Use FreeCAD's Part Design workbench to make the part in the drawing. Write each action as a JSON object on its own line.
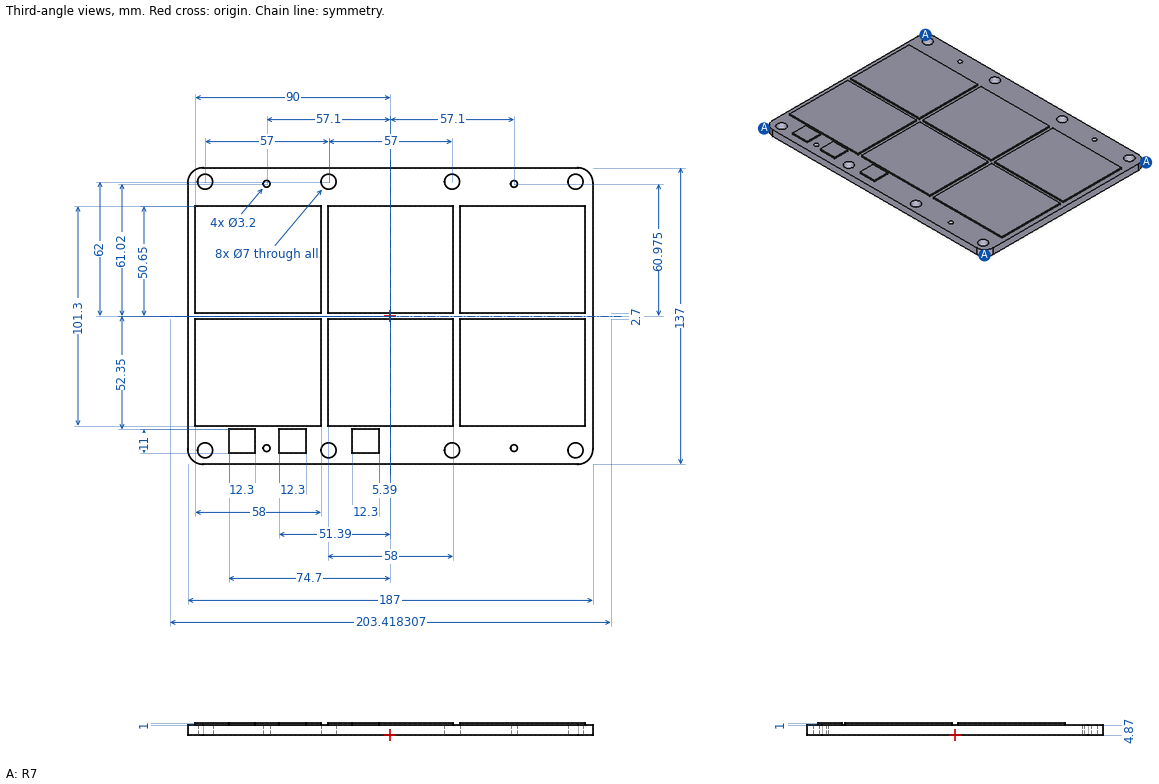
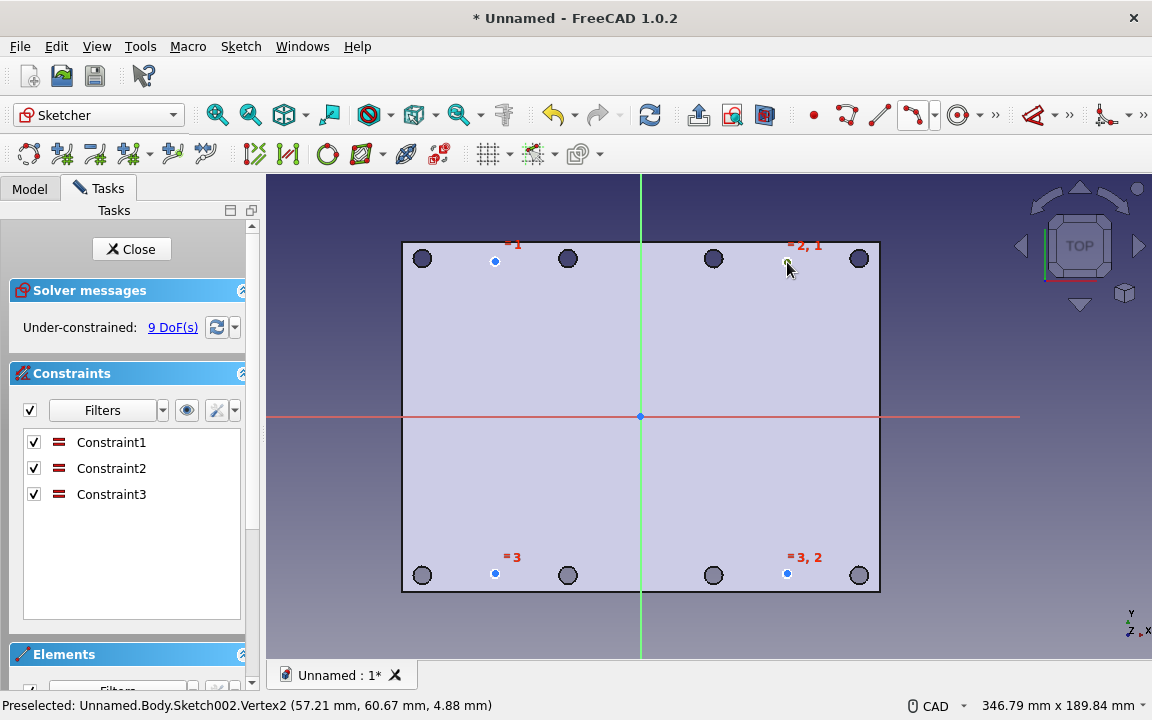
{"action": "left_click", "coordinate": [787, 574]}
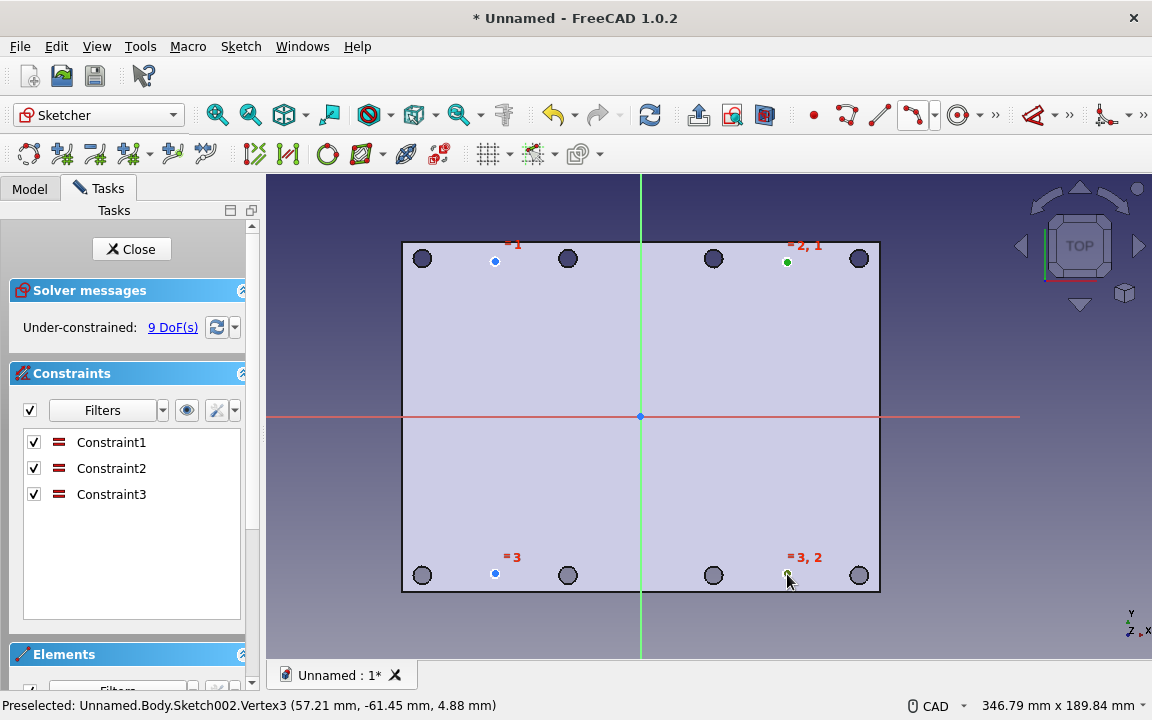
{"action": "left_click", "coordinate": [344, 417]}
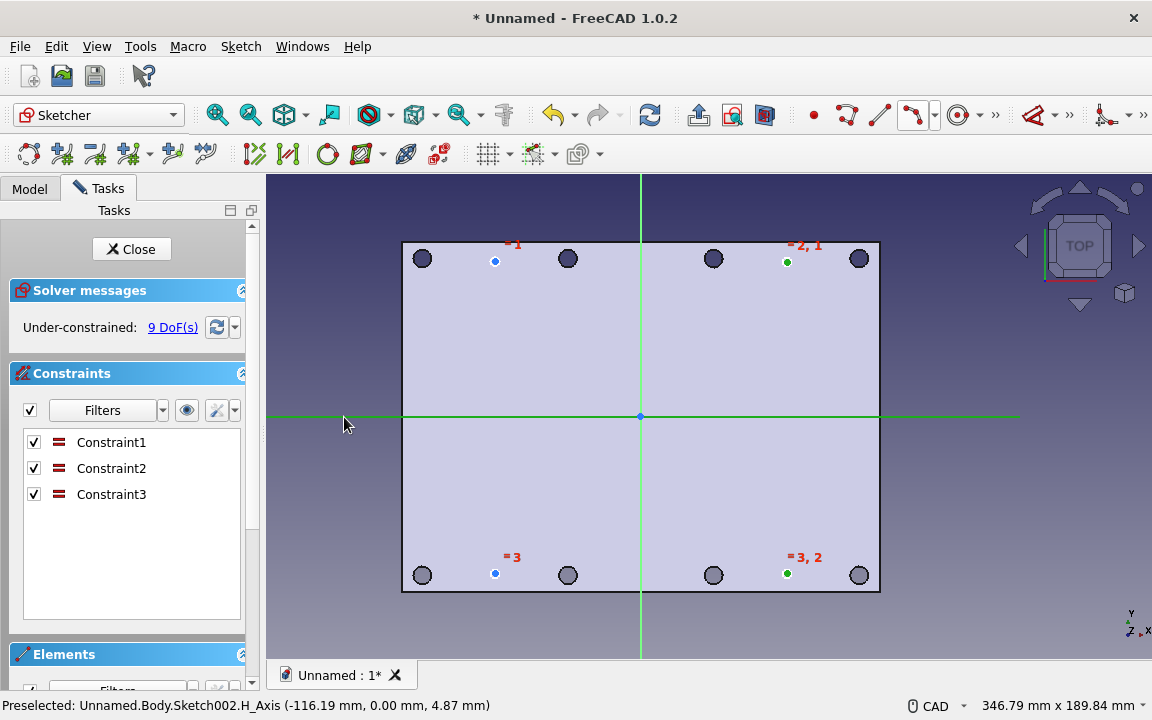
{"action": "key", "text": "s"}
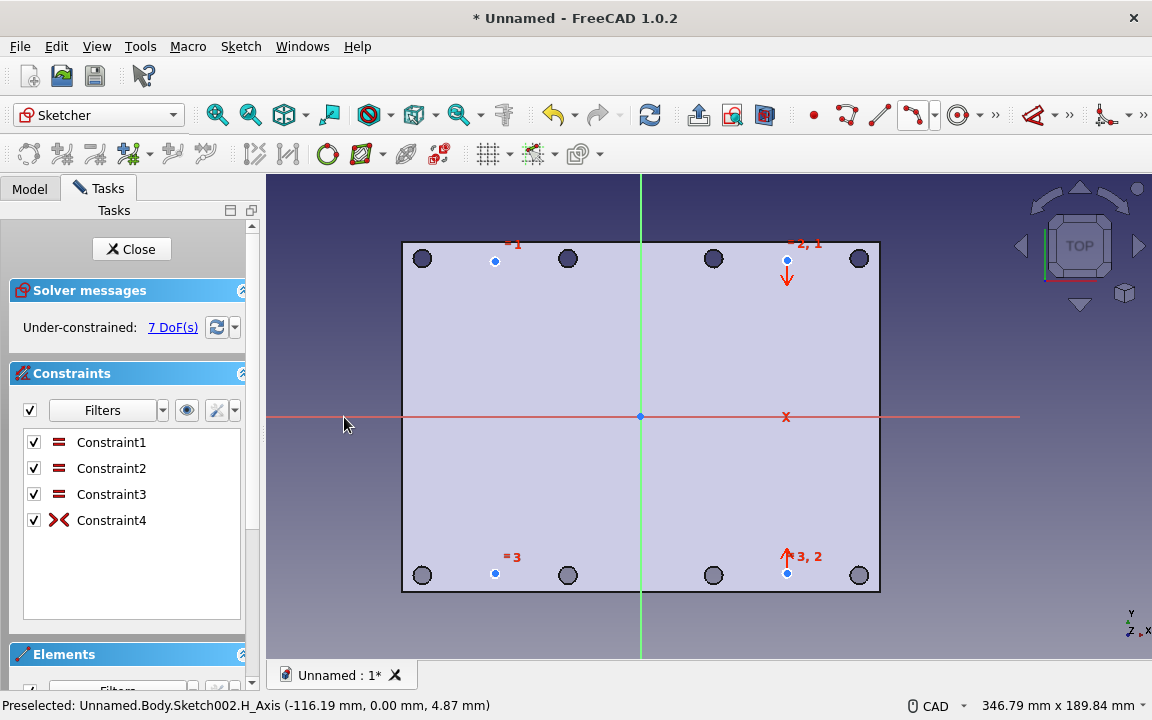
{"action": "left_click", "coordinate": [495, 262]}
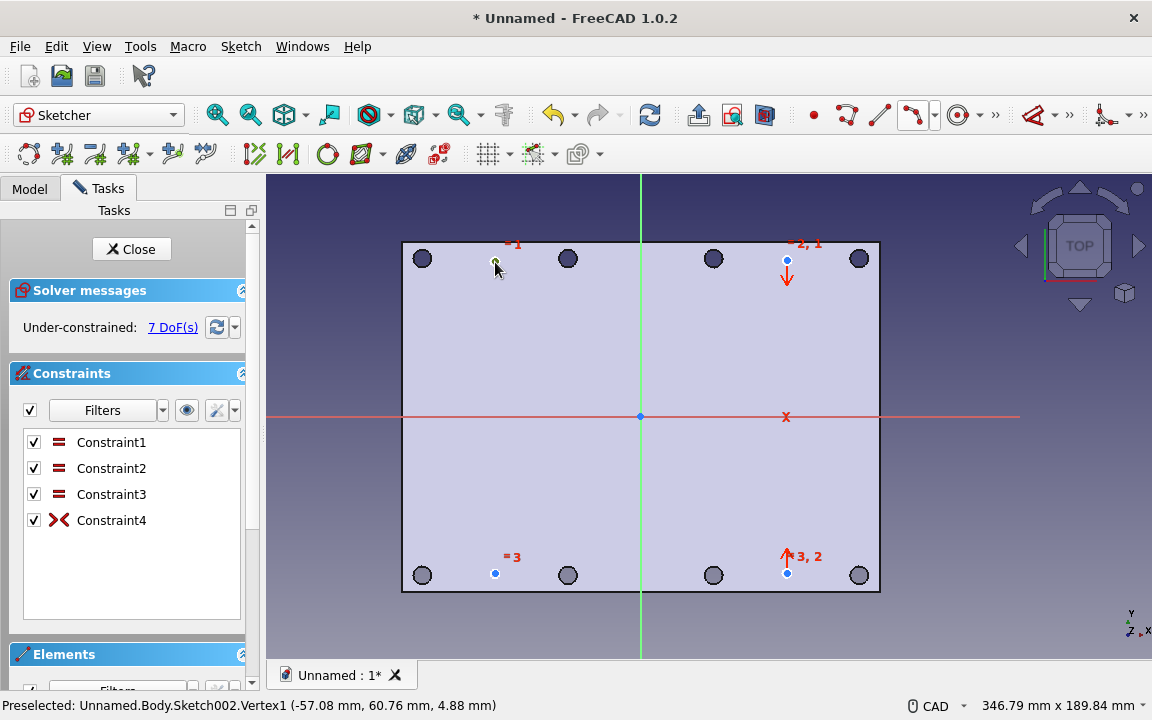
{"action": "left_click", "coordinate": [495, 574]}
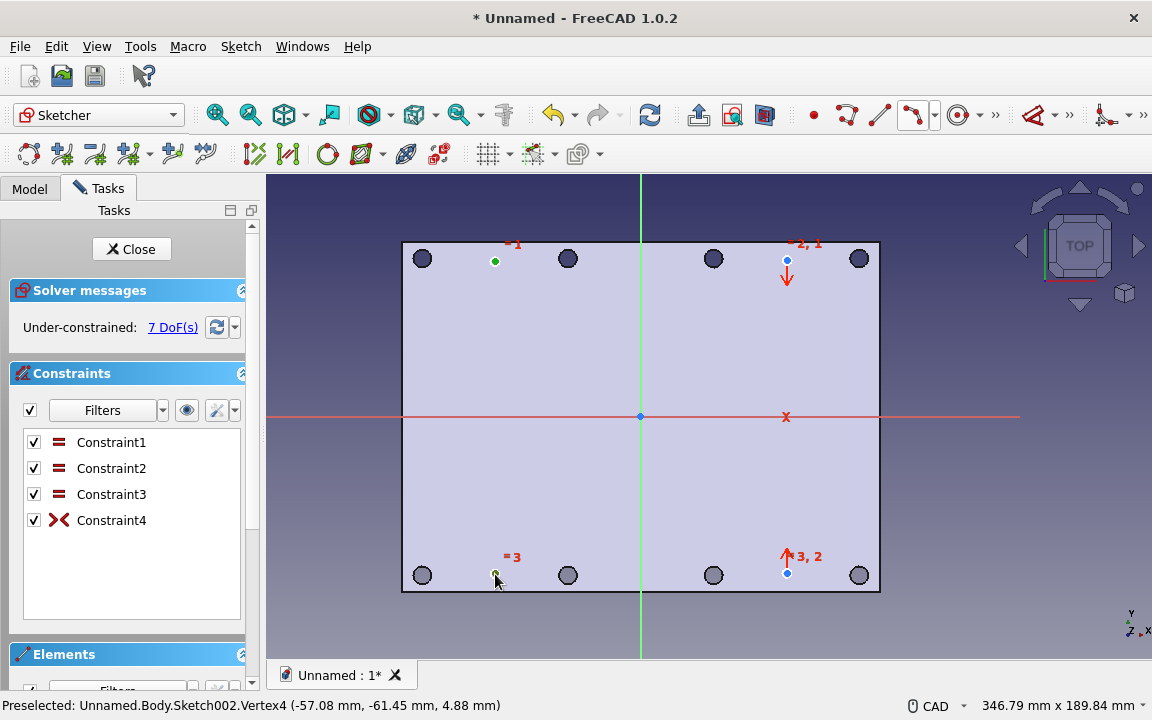
{"action": "left_click", "coordinate": [344, 417]}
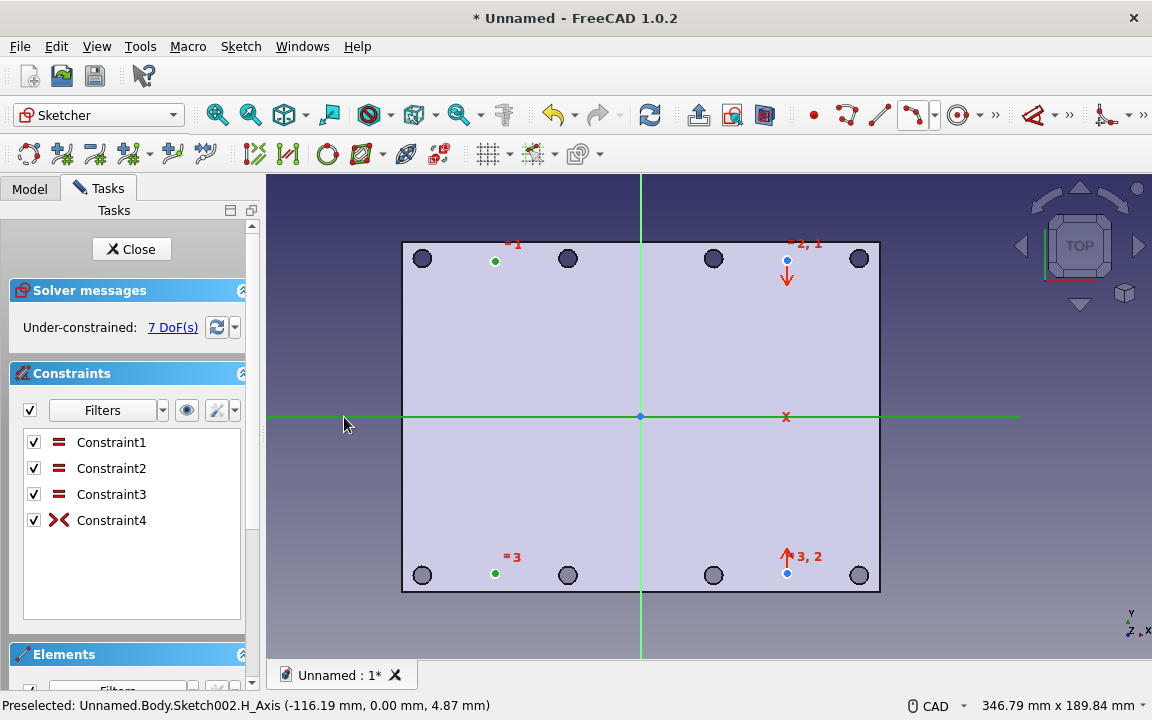
{"action": "key", "text": "s"}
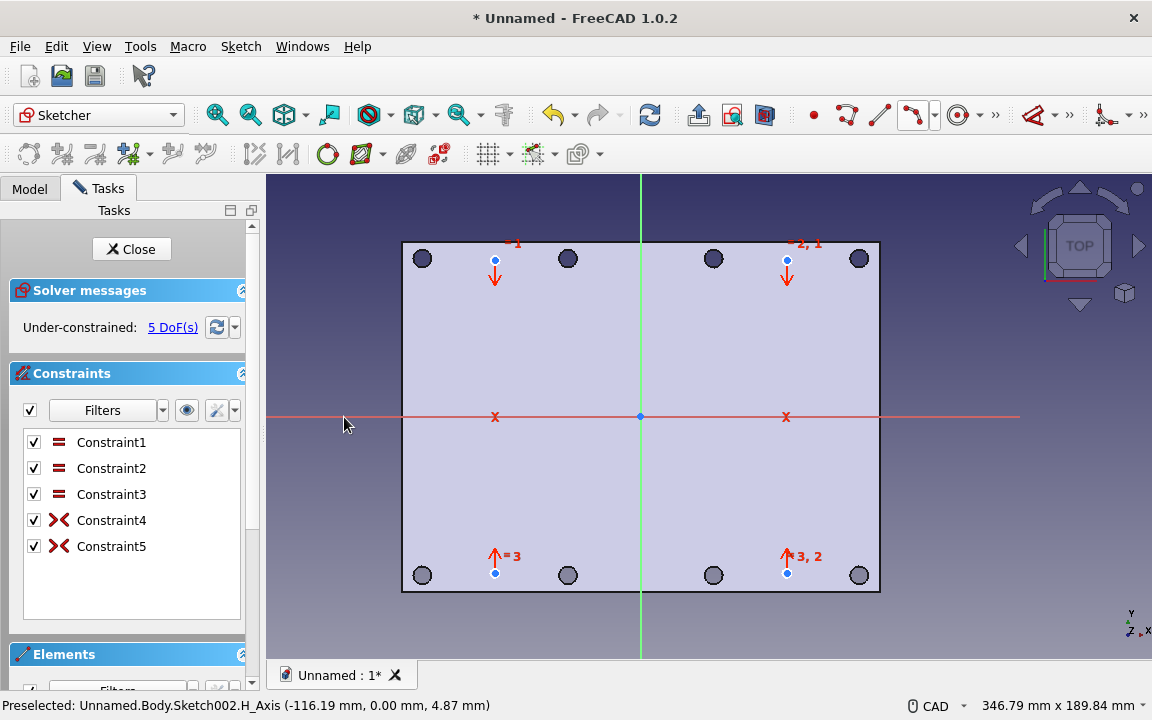
{"action": "key", "text": "d"}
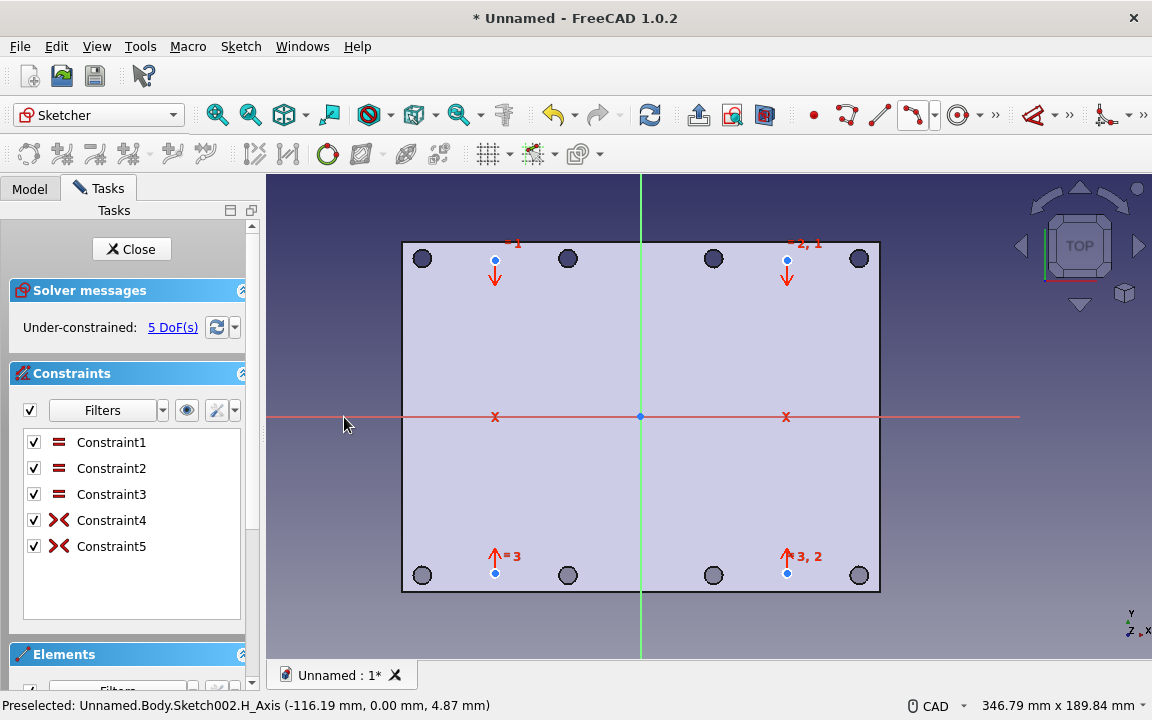
{"action": "scroll", "coordinate": [495, 256], "scroll_direction": "up", "scroll_amount": 8}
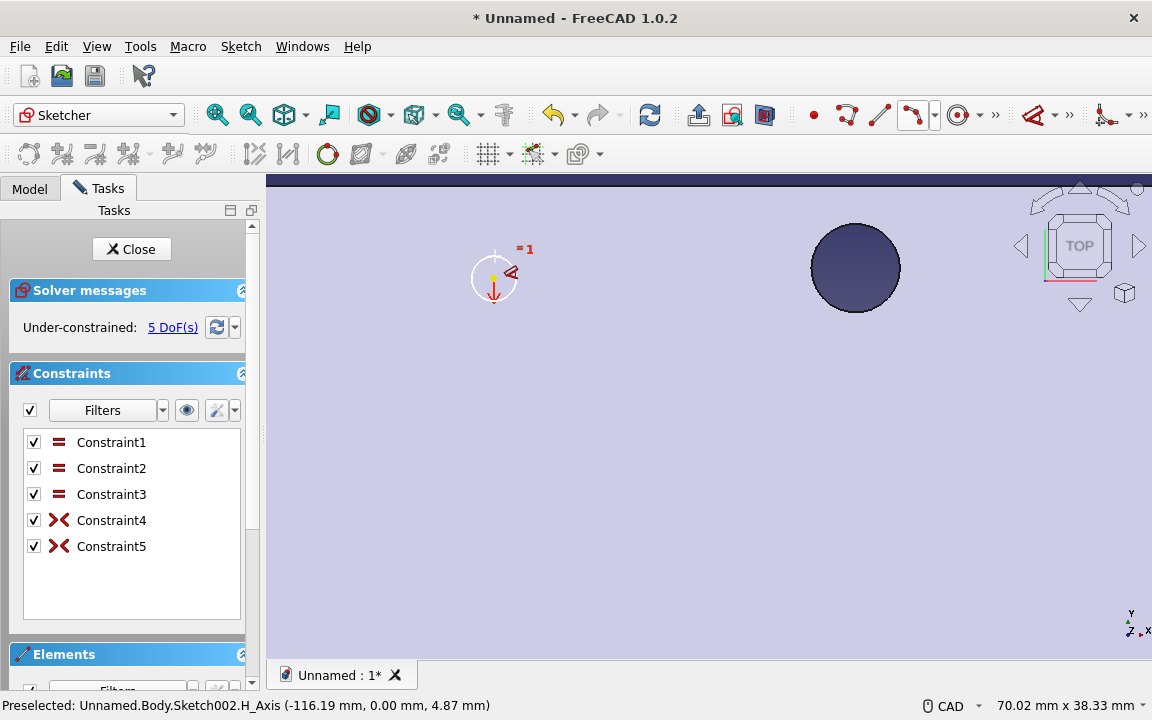
{"action": "left_click", "coordinate": [495, 256]}
{"action": "left_click", "coordinate": [496, 224]}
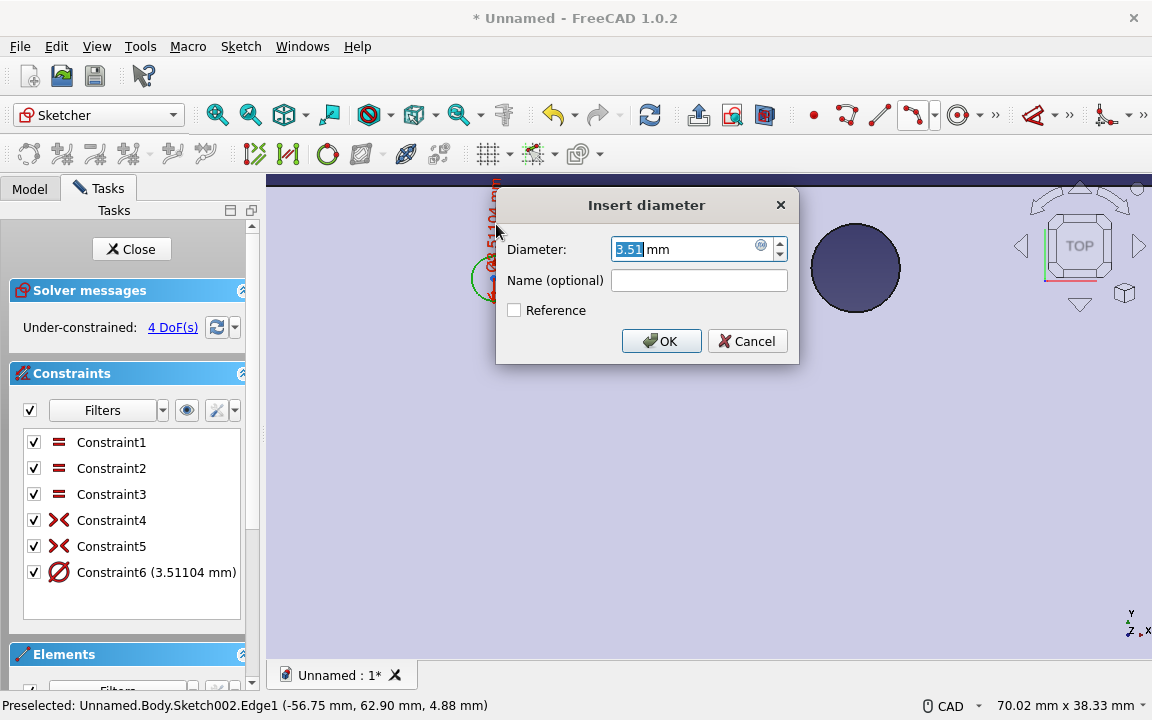
{"action": "type", "text": "3.2"}
{"action": "key", "text": "Return"}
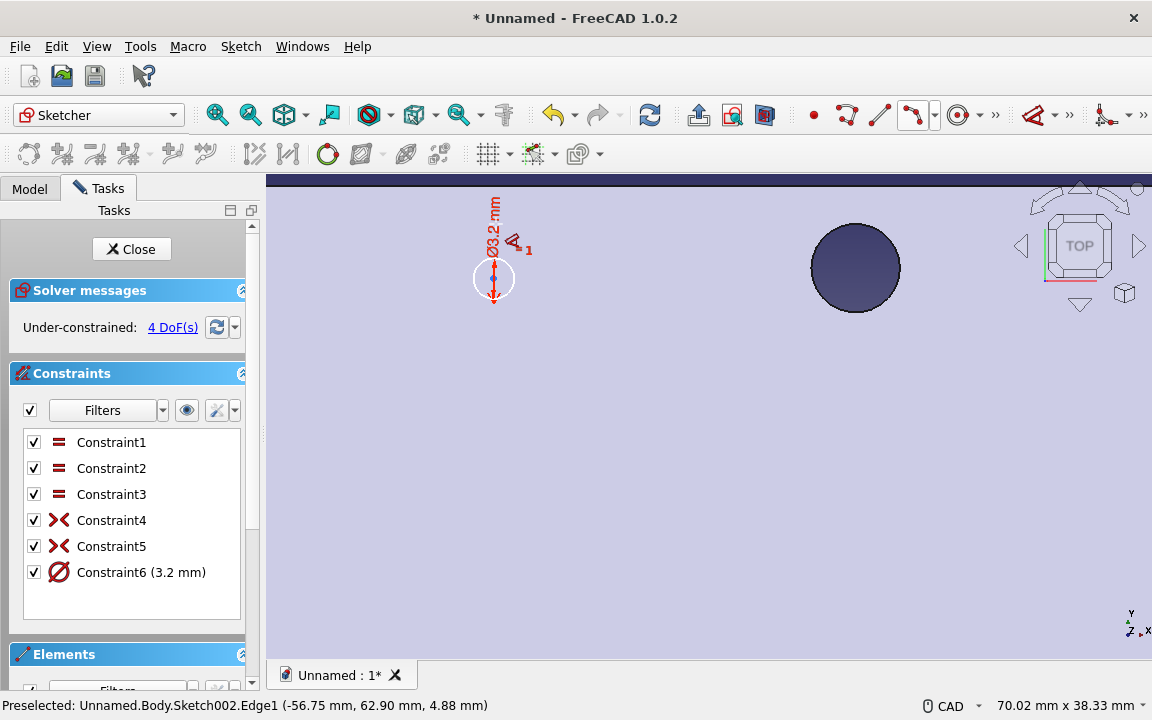
{"action": "scroll", "coordinate": [495, 256], "scroll_direction": "down", "scroll_amount": 8}